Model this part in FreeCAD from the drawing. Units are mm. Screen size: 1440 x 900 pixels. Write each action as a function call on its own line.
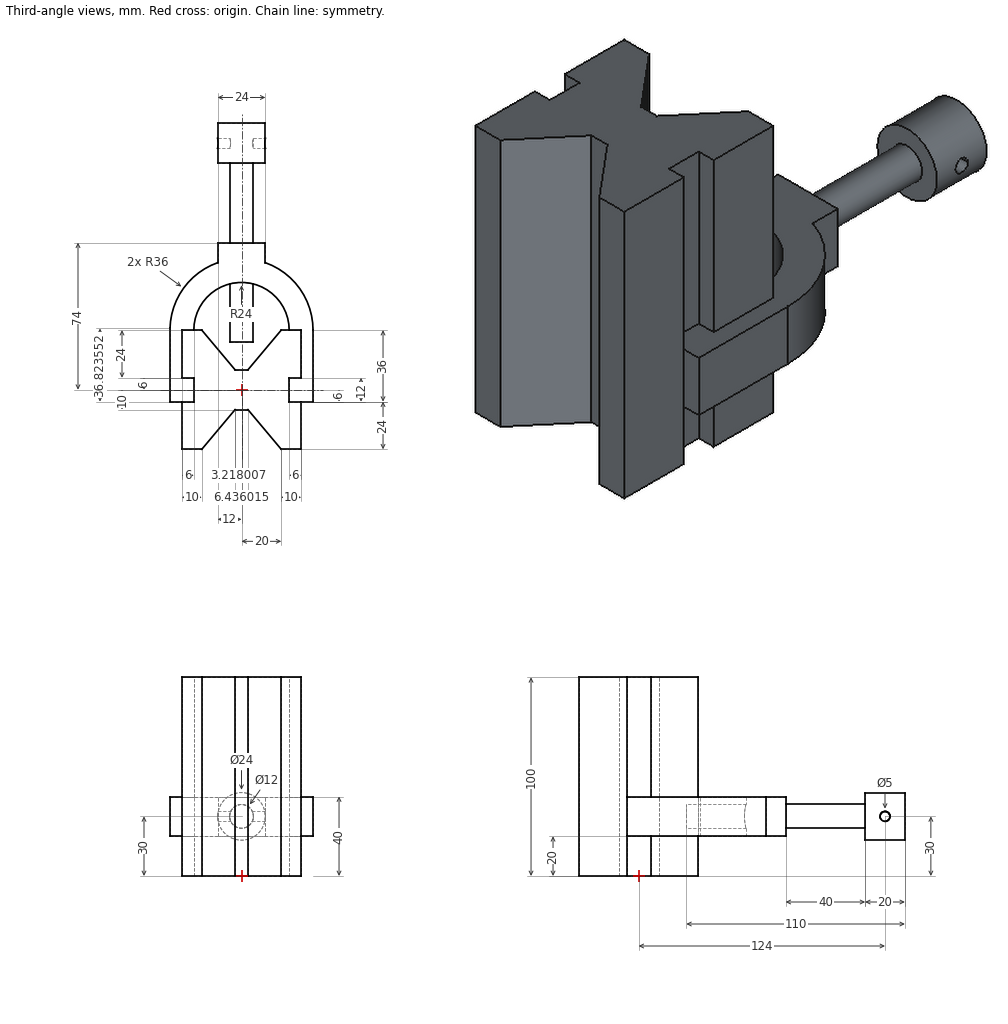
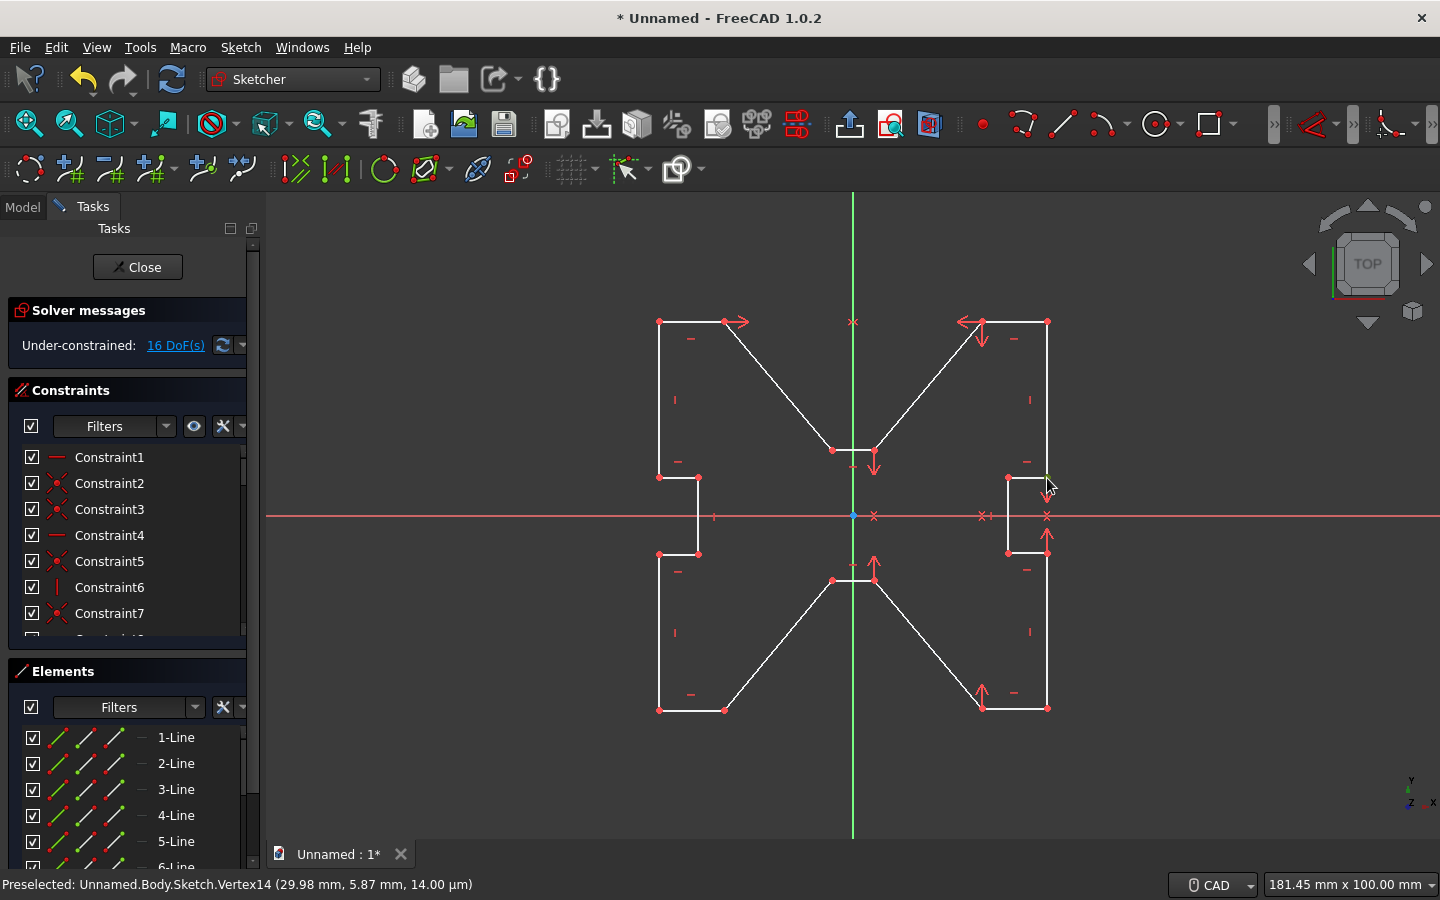
click(659, 478)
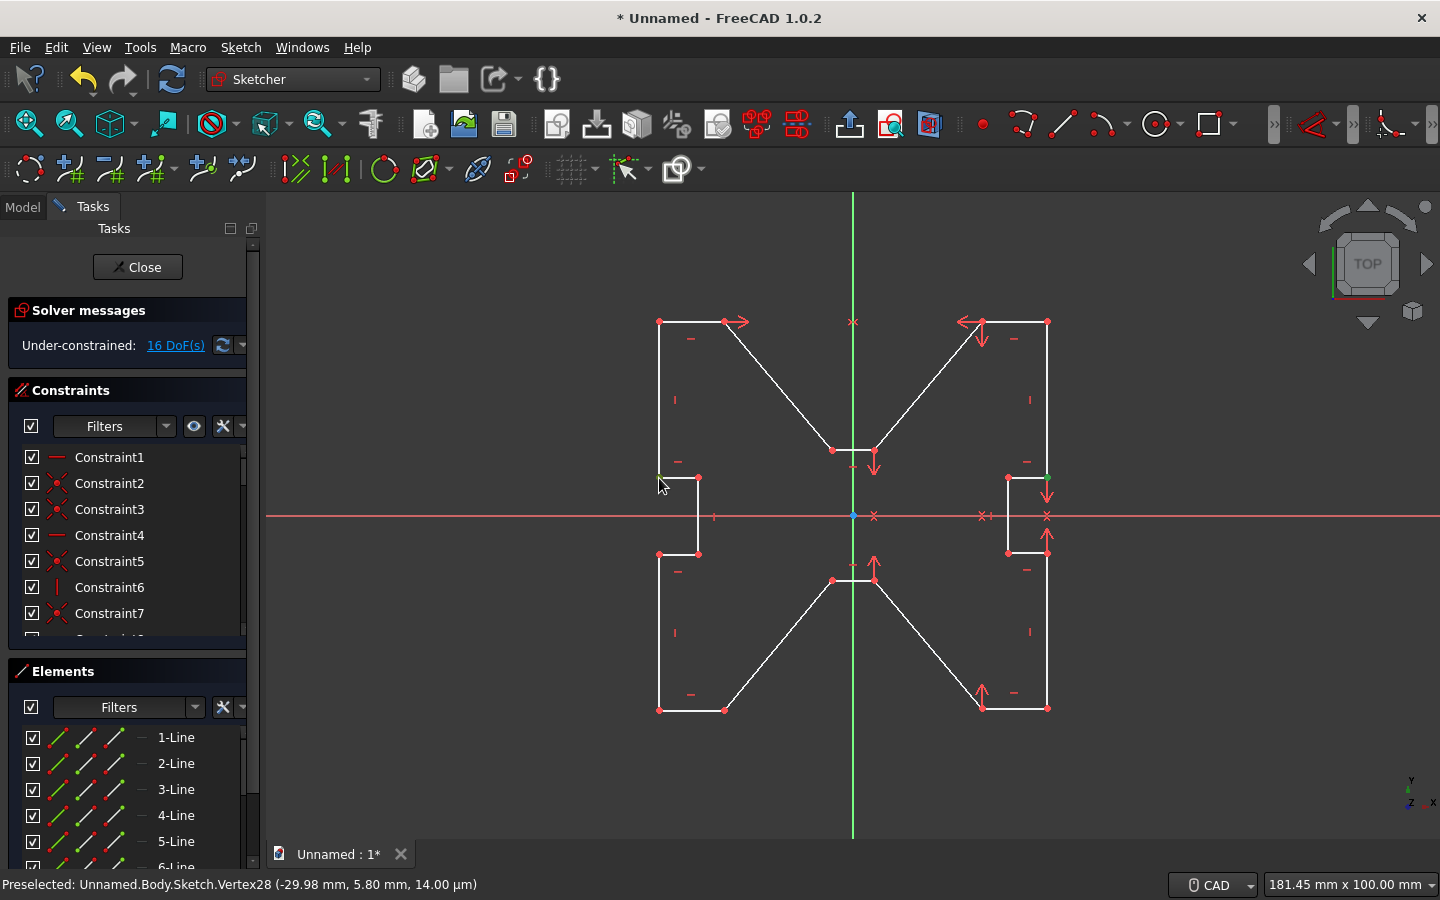
click(853, 769)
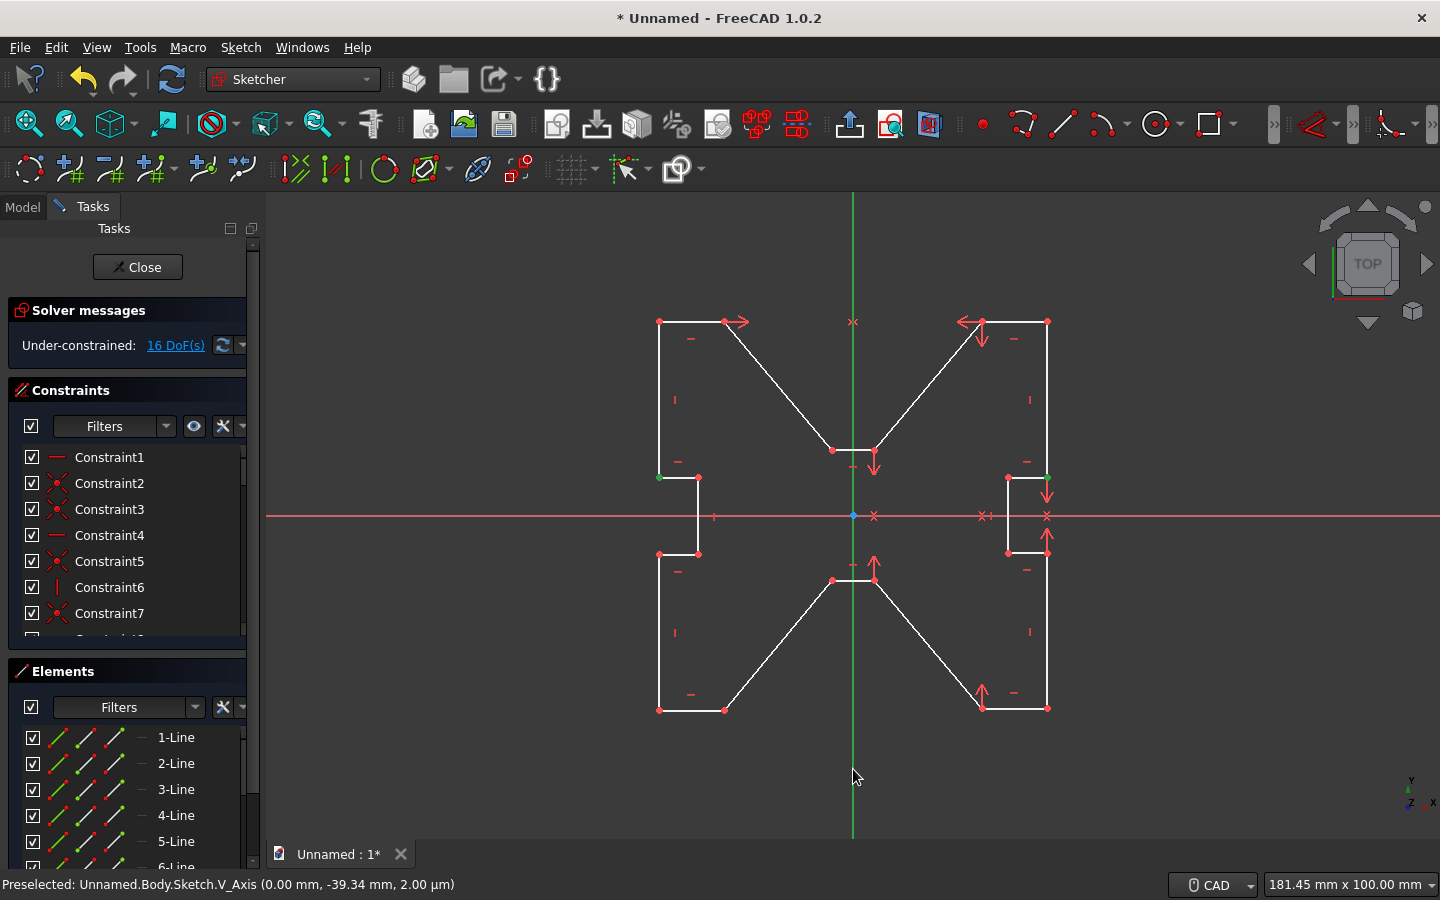
key(s)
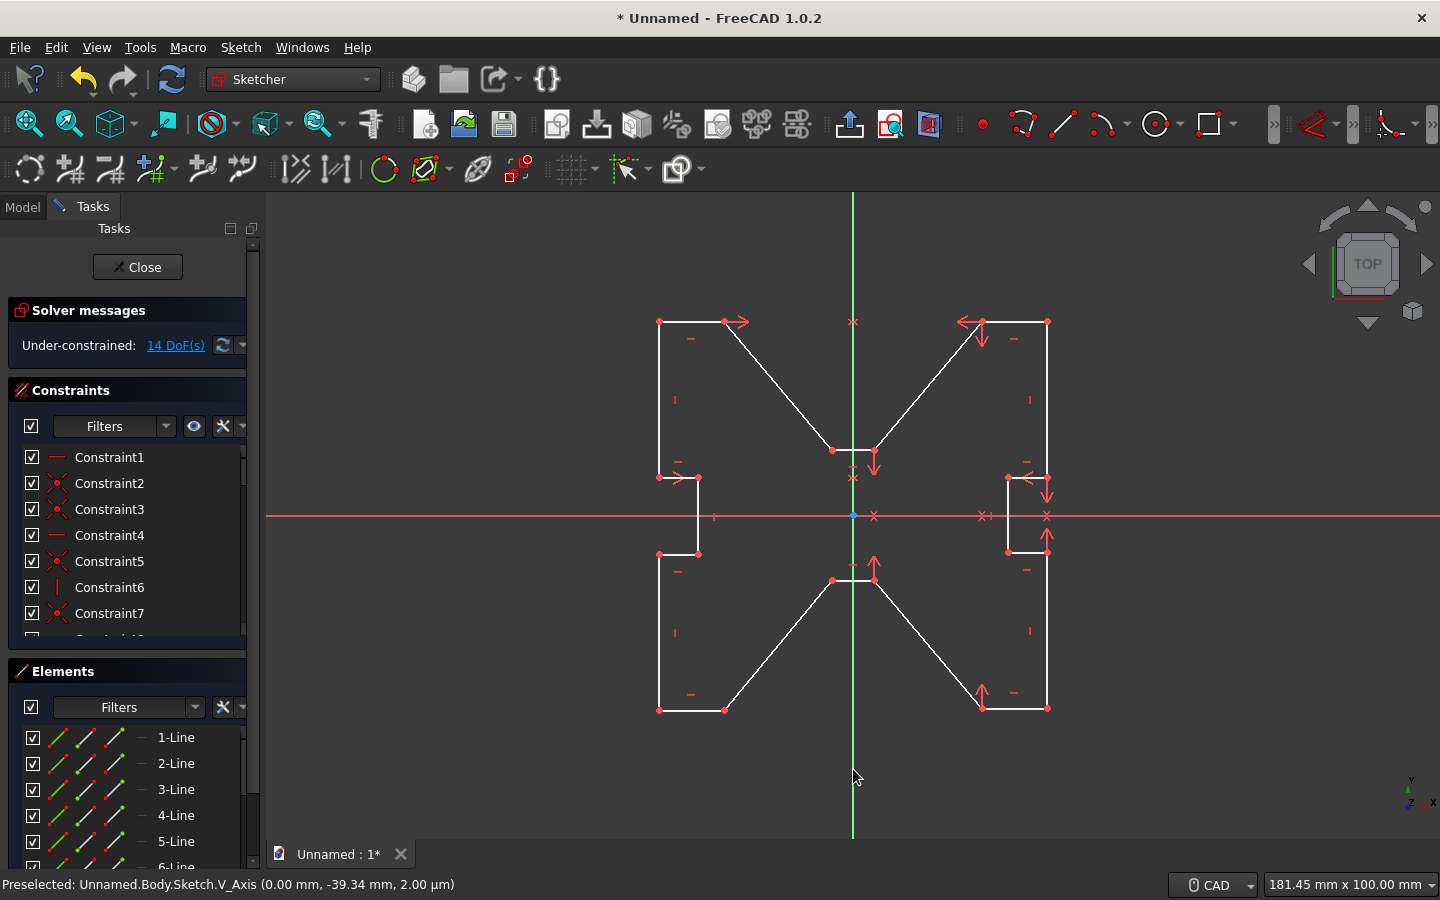
click(1008, 553)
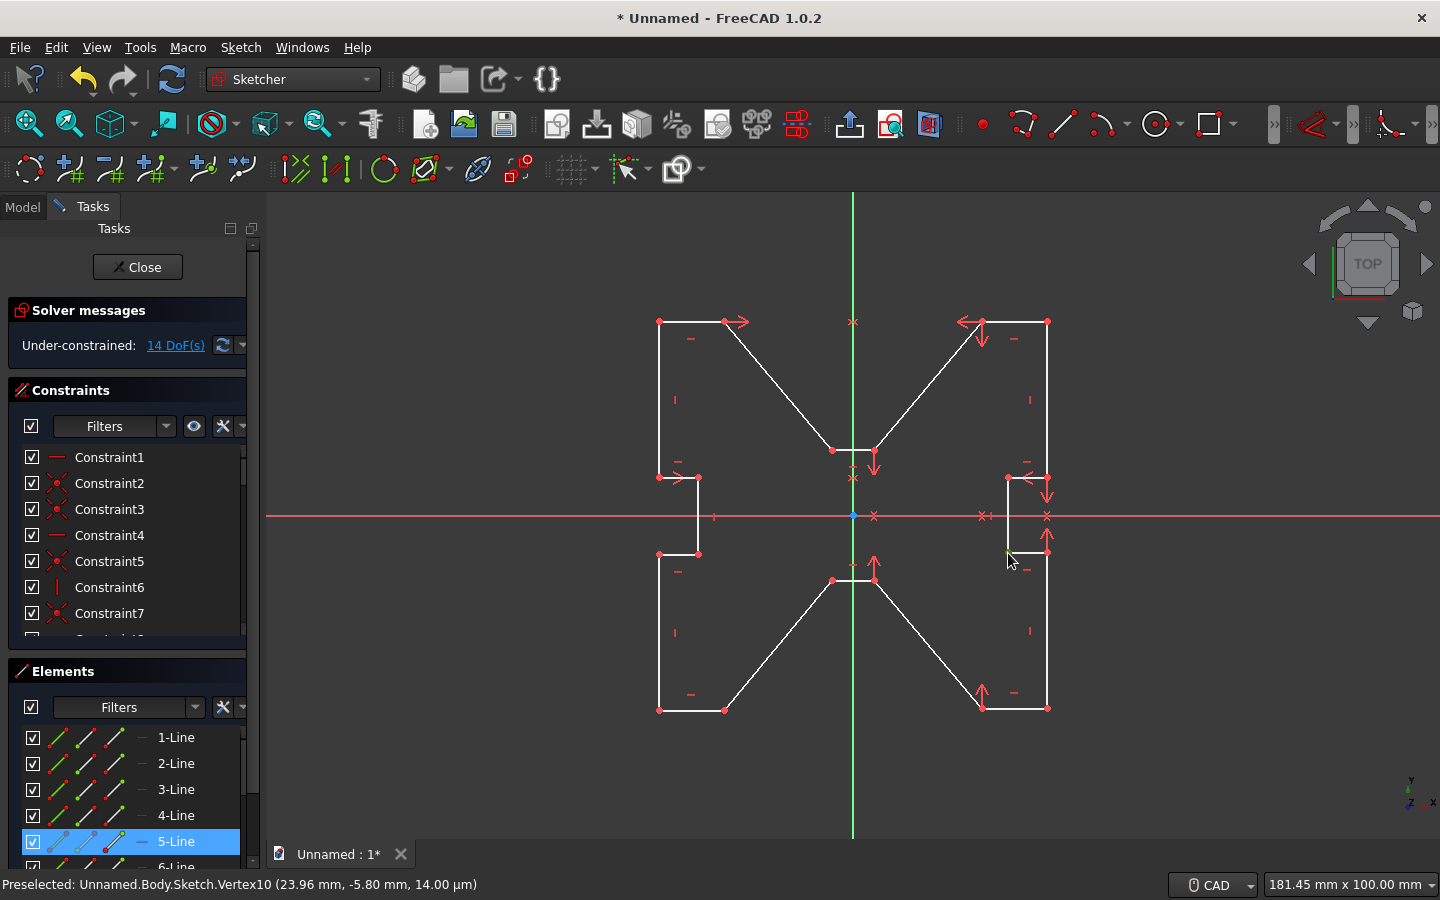
click(698, 555)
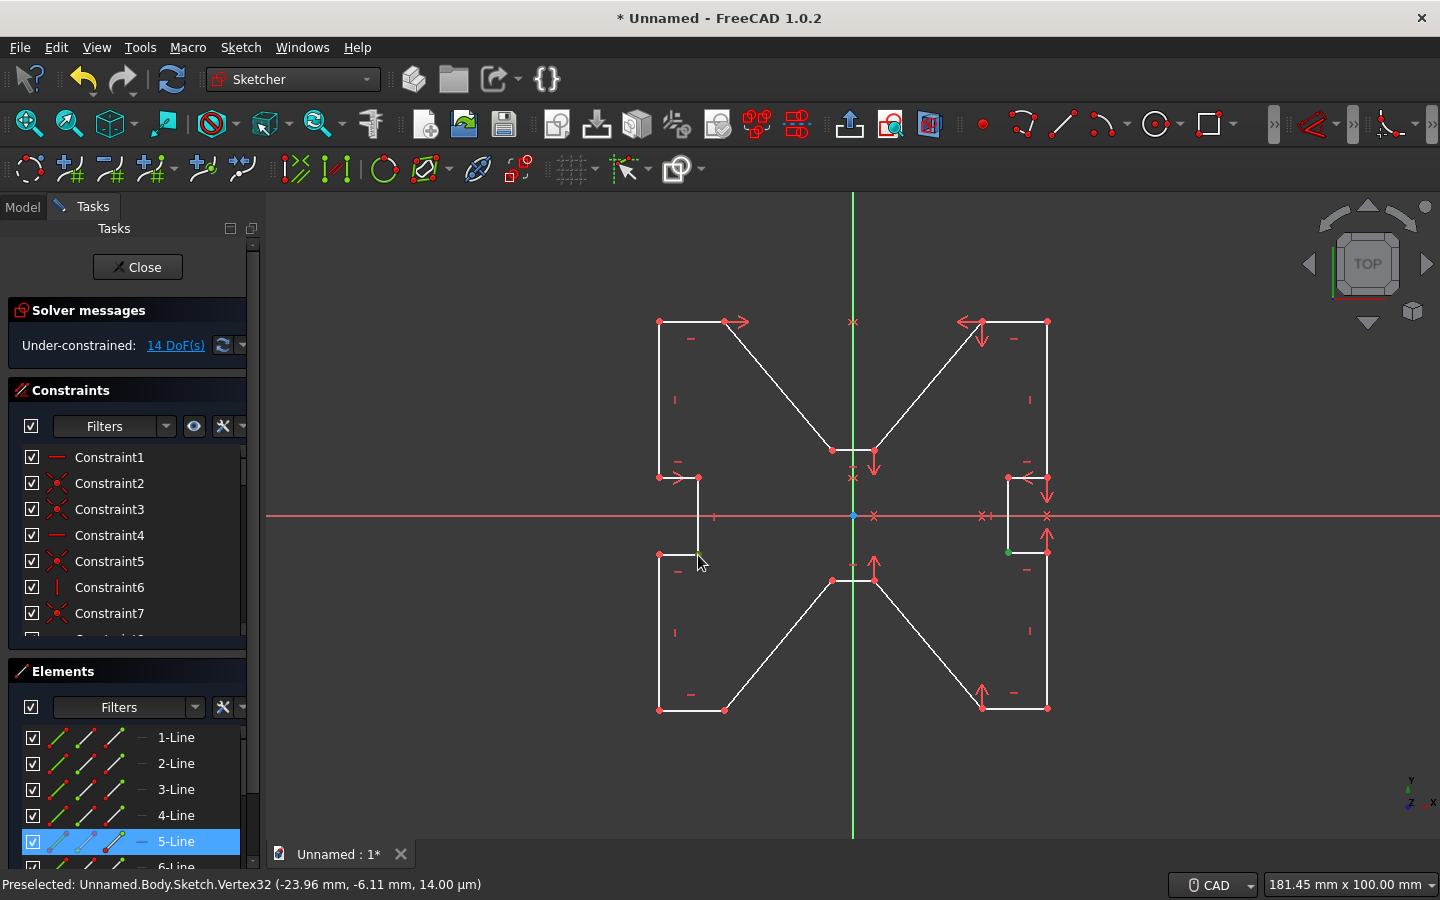
click(853, 769)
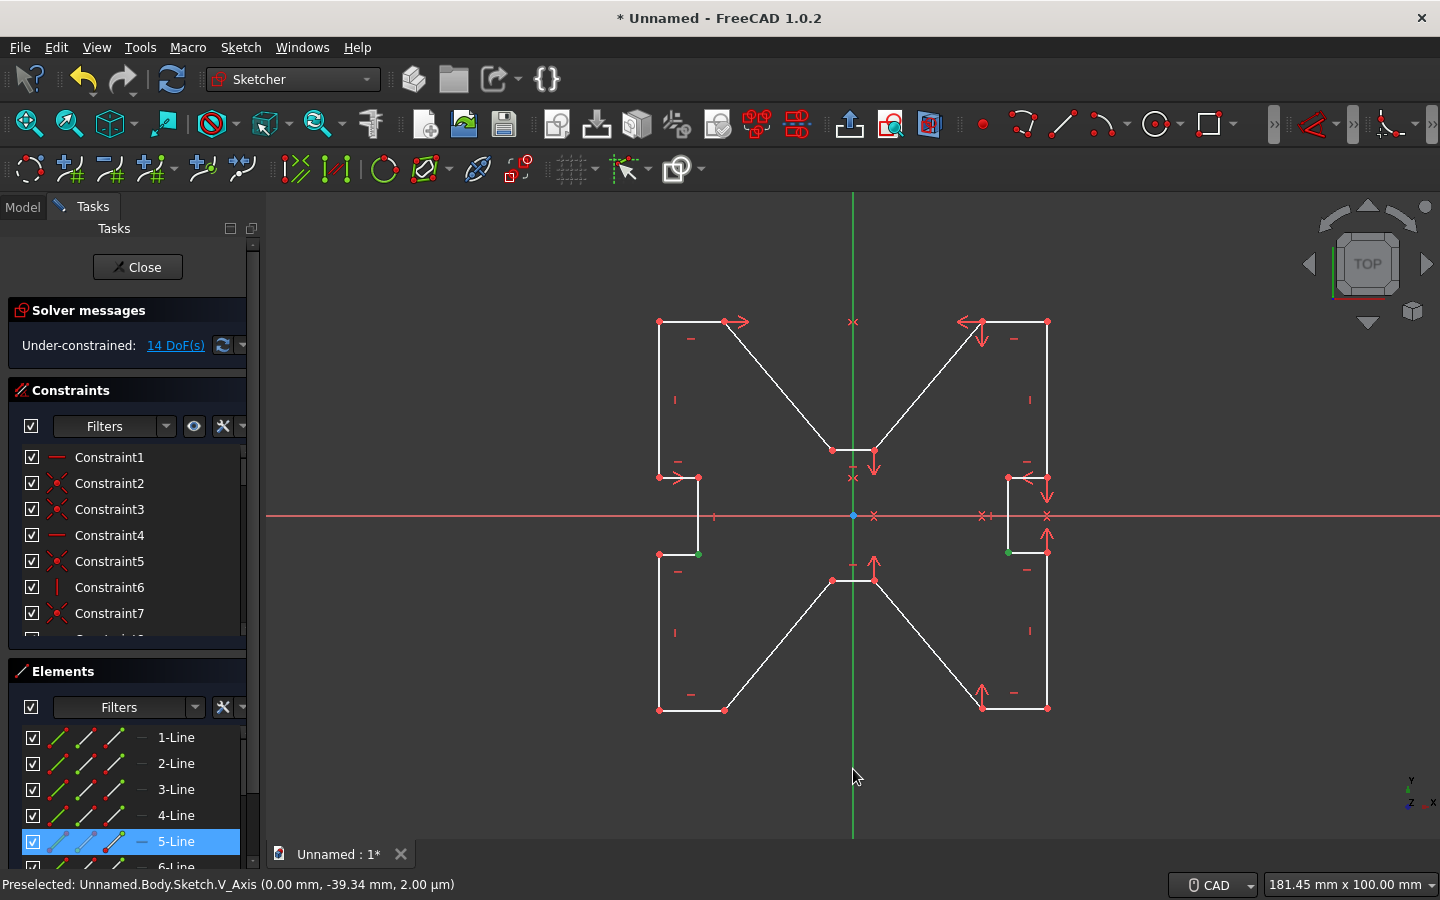
key(s)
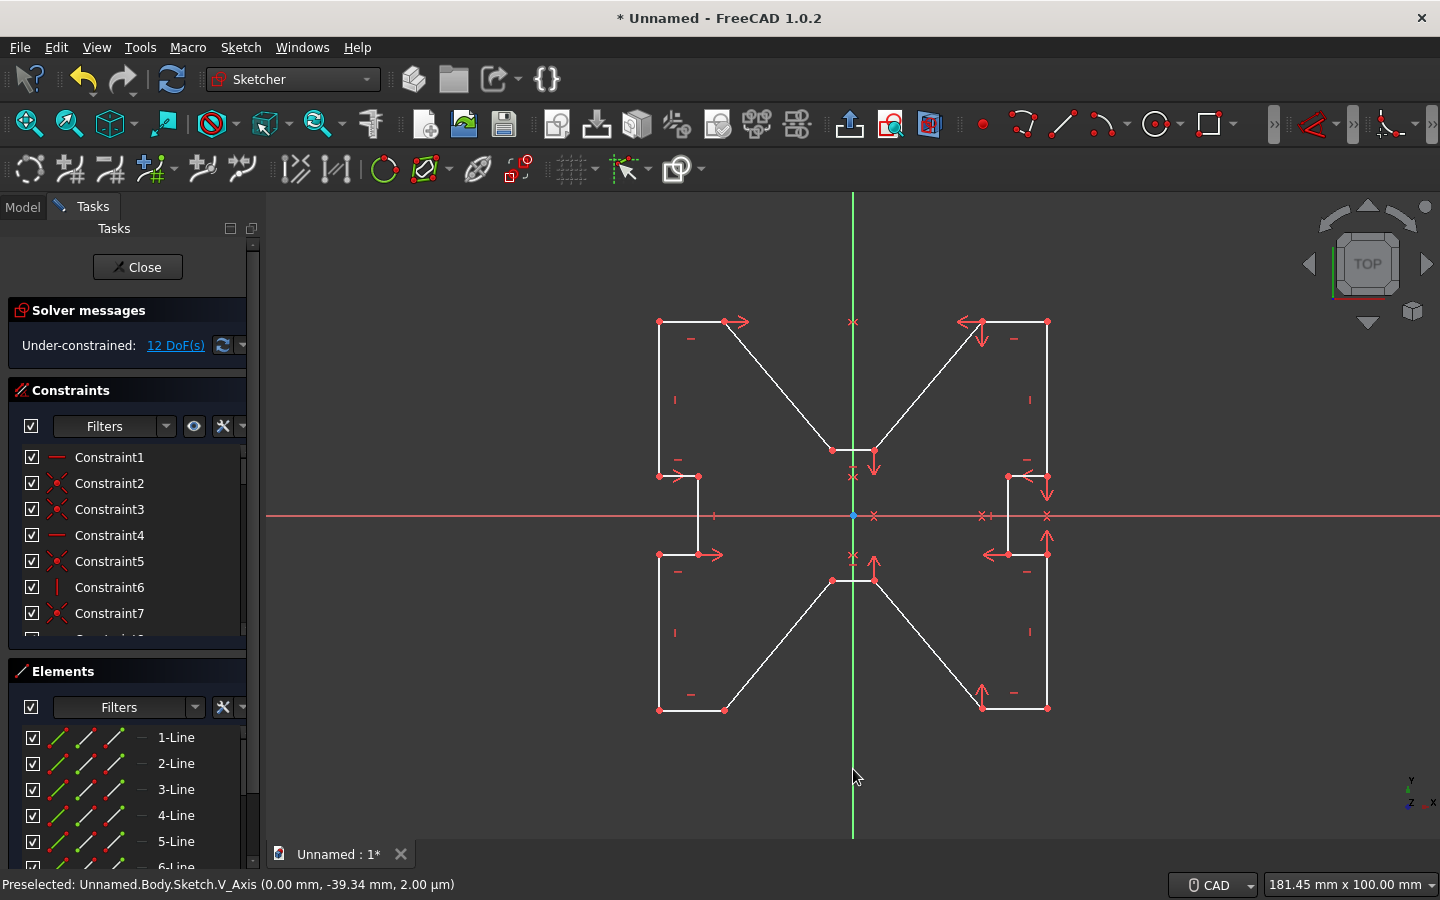
click(1047, 709)